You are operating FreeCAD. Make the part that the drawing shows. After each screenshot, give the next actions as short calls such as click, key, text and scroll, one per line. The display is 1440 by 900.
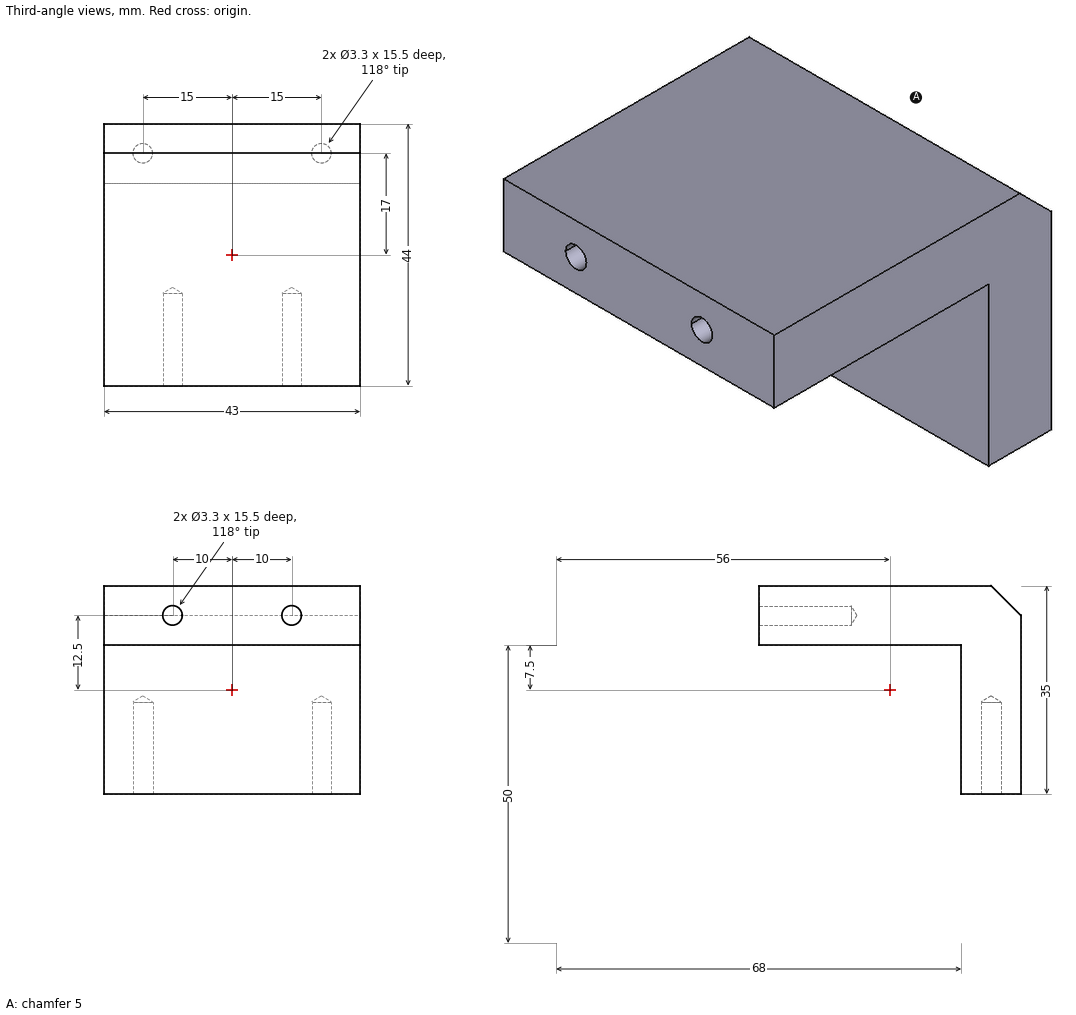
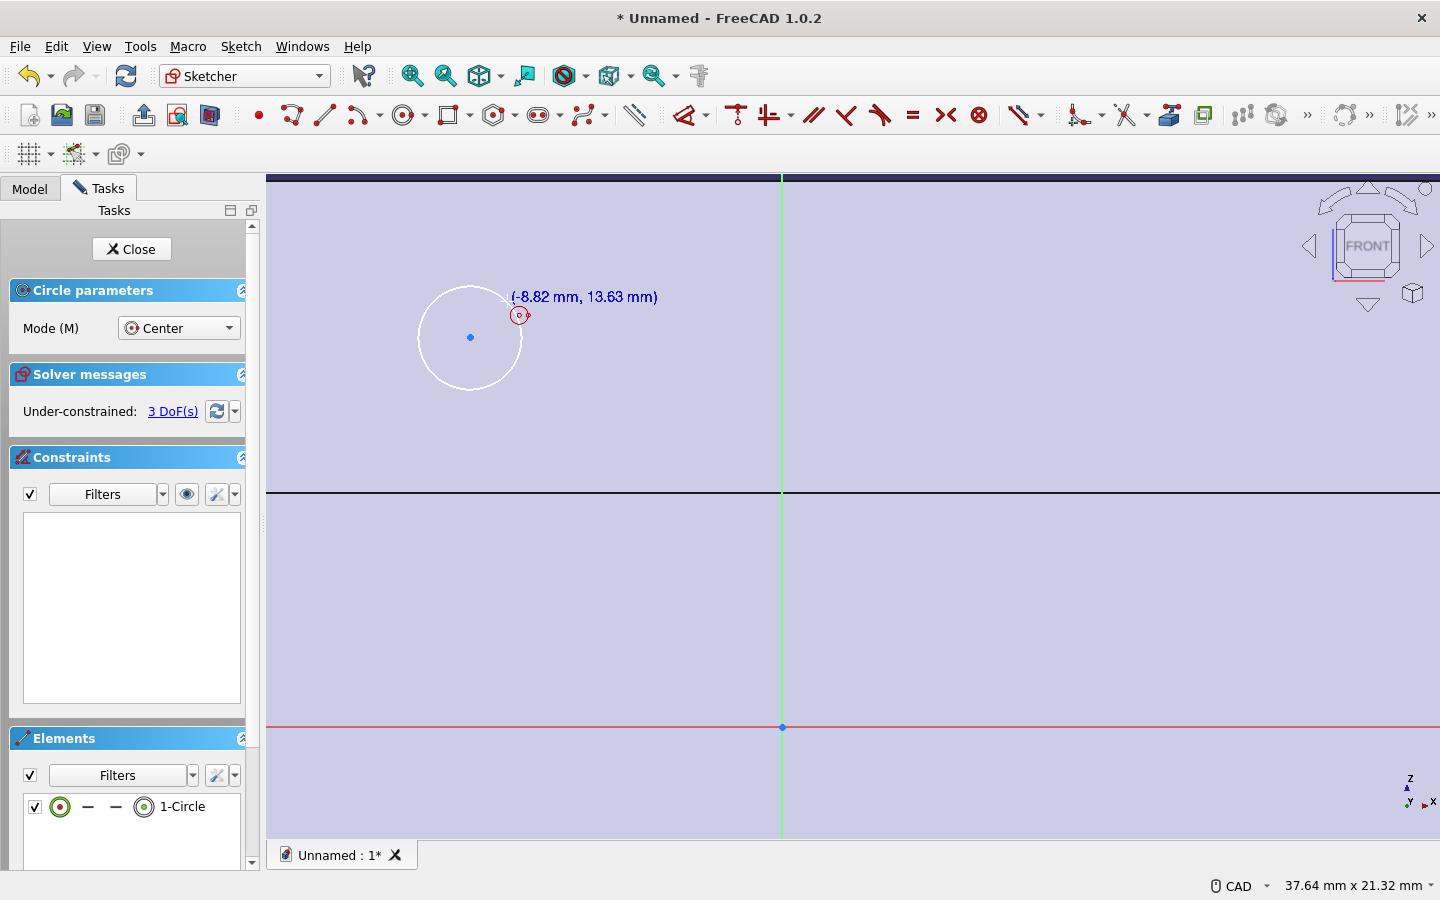
click(1094, 337)
click(1130, 301)
key(Escape)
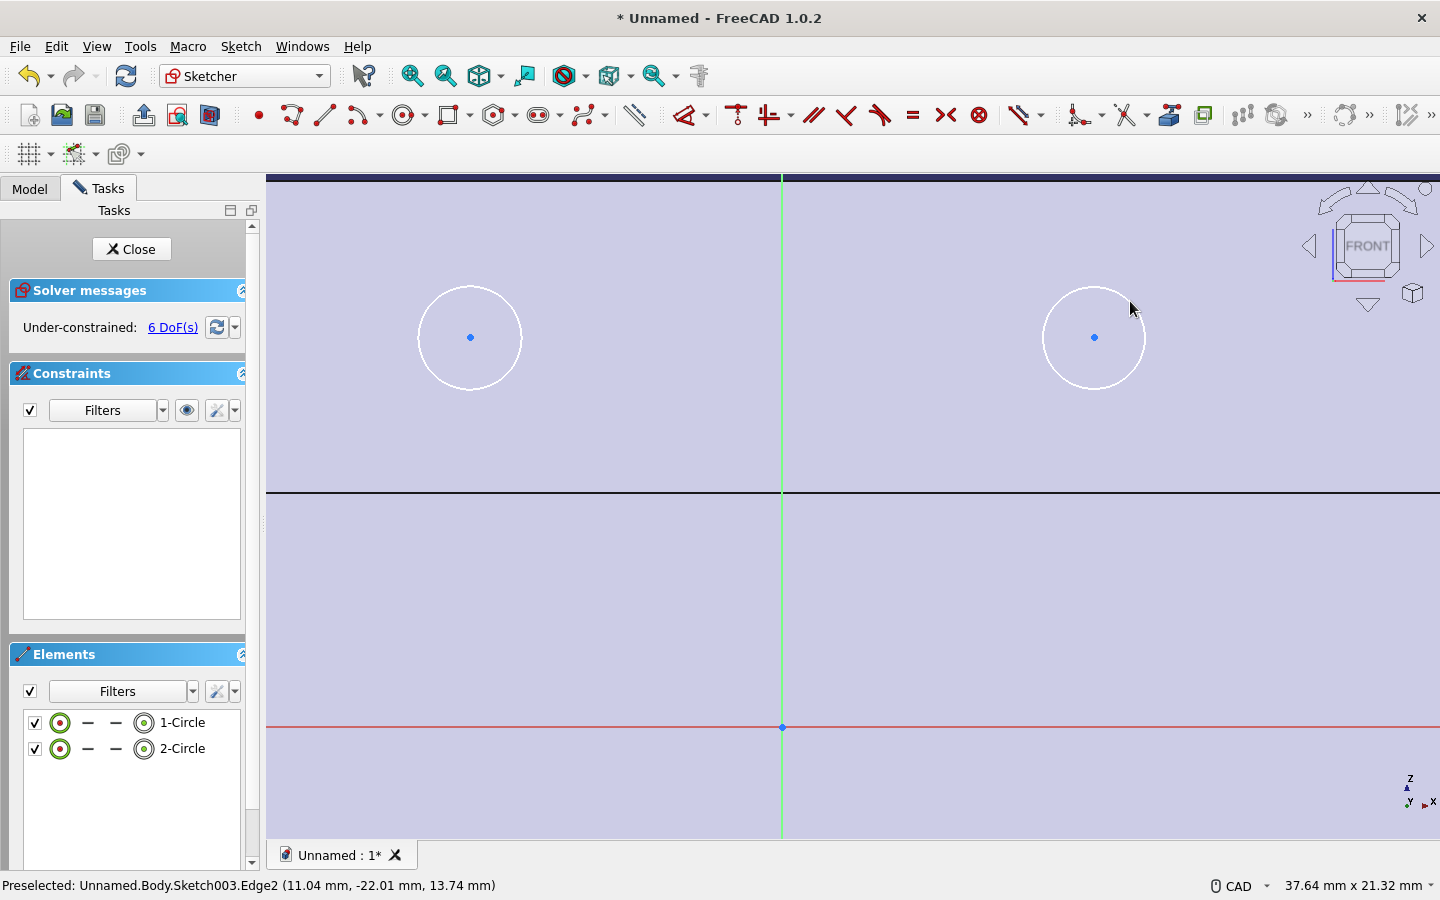
click(506, 301)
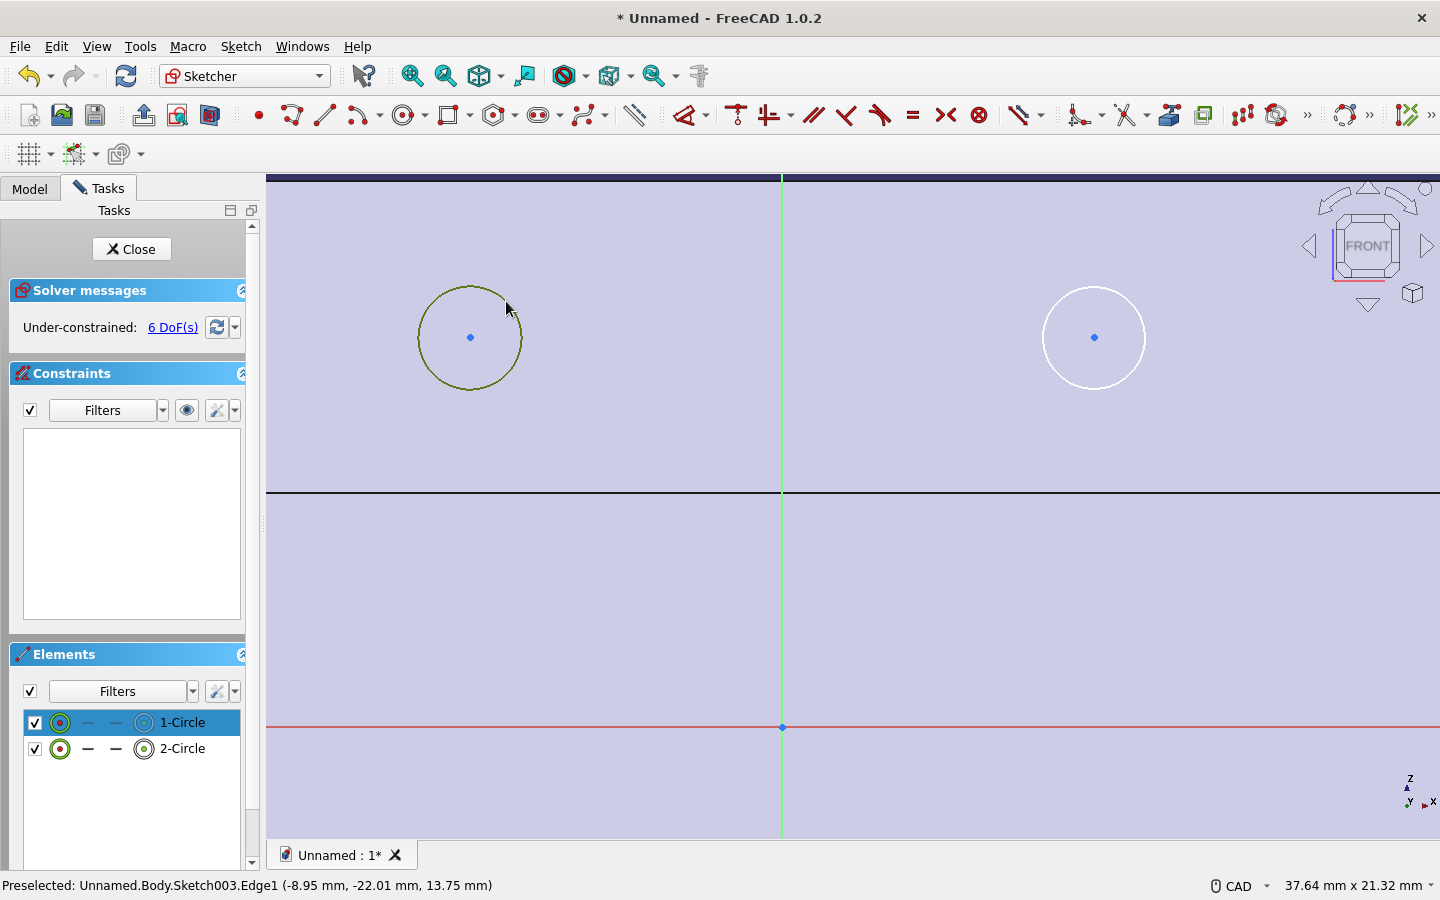
click(1130, 302)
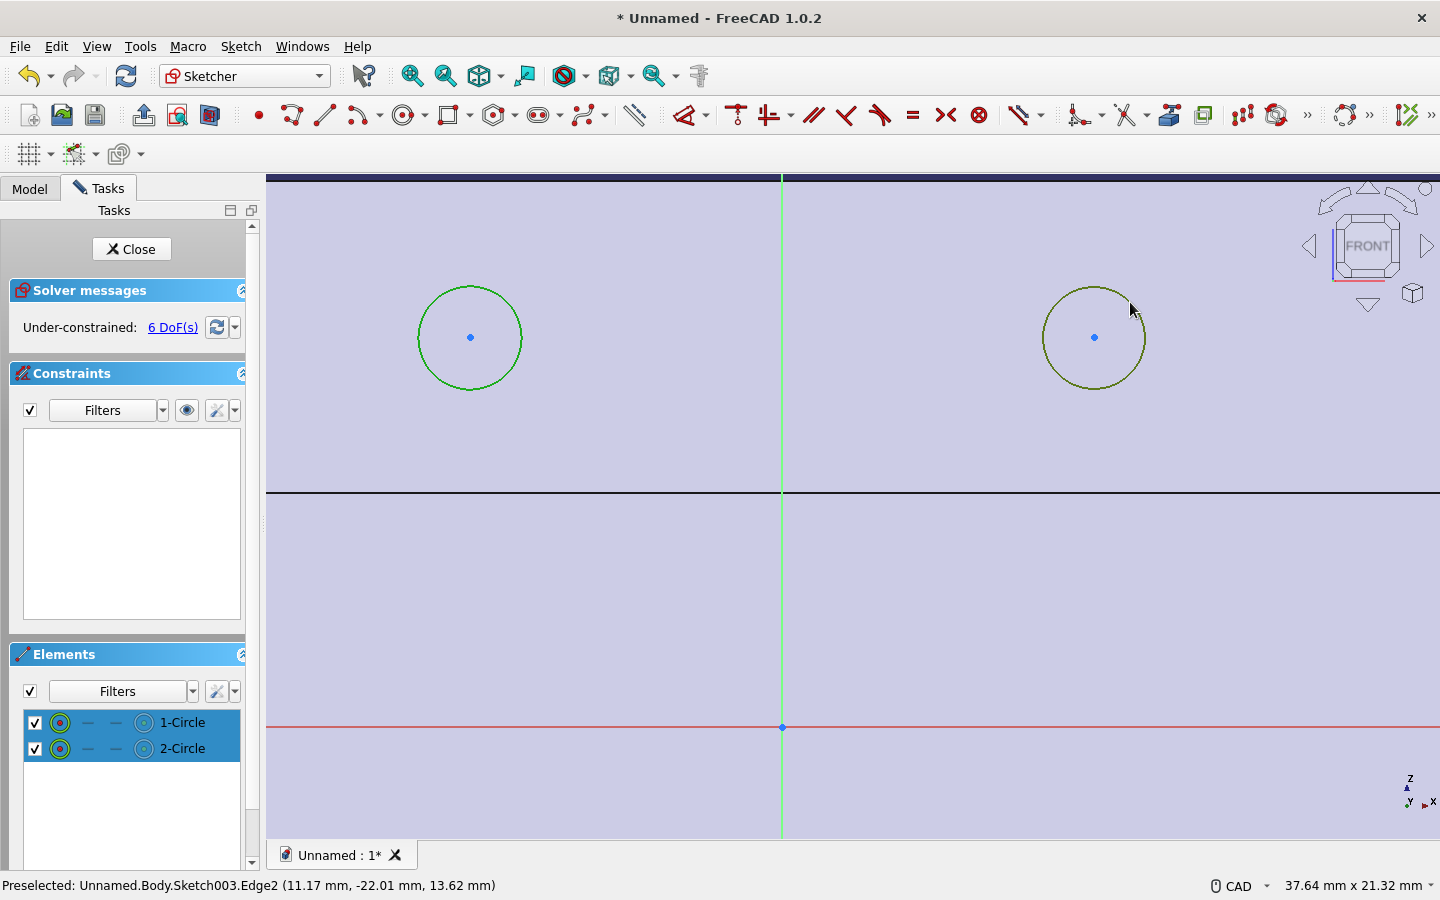
click(913, 116)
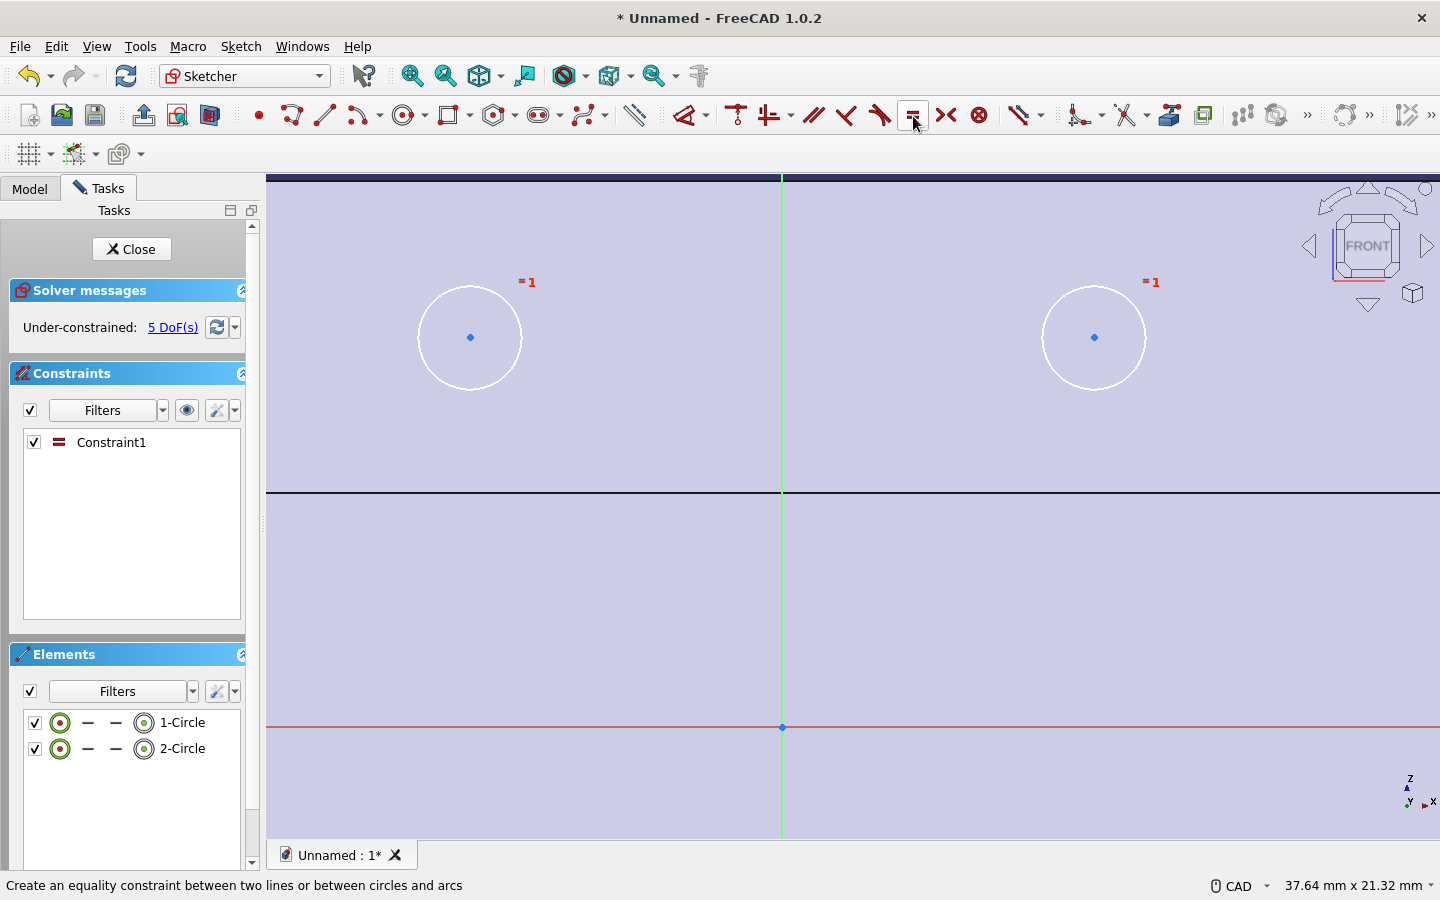
click(684, 116)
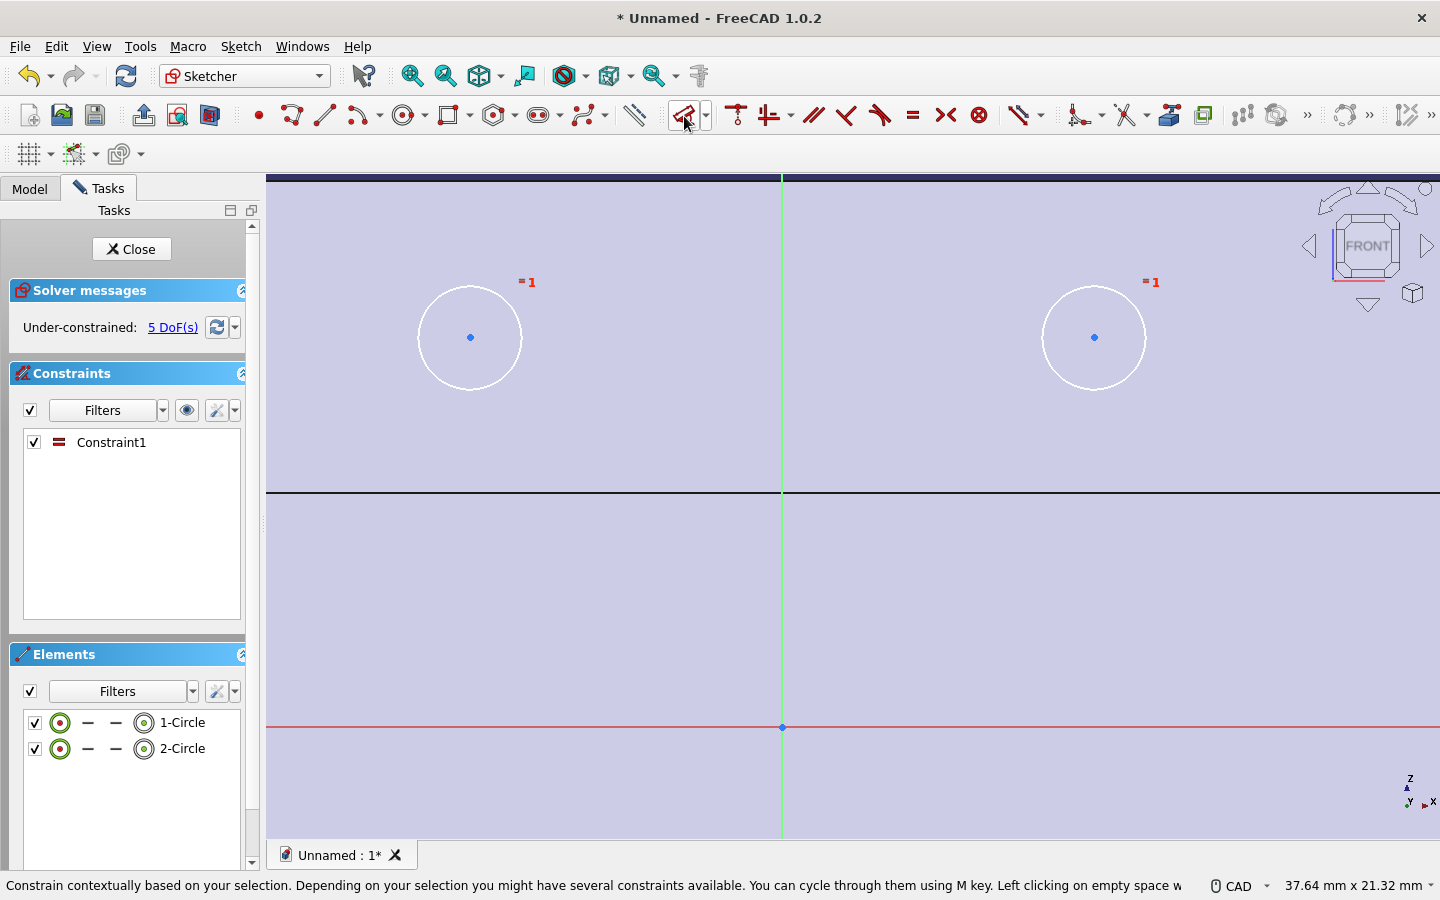
click(506, 301)
click(528, 278)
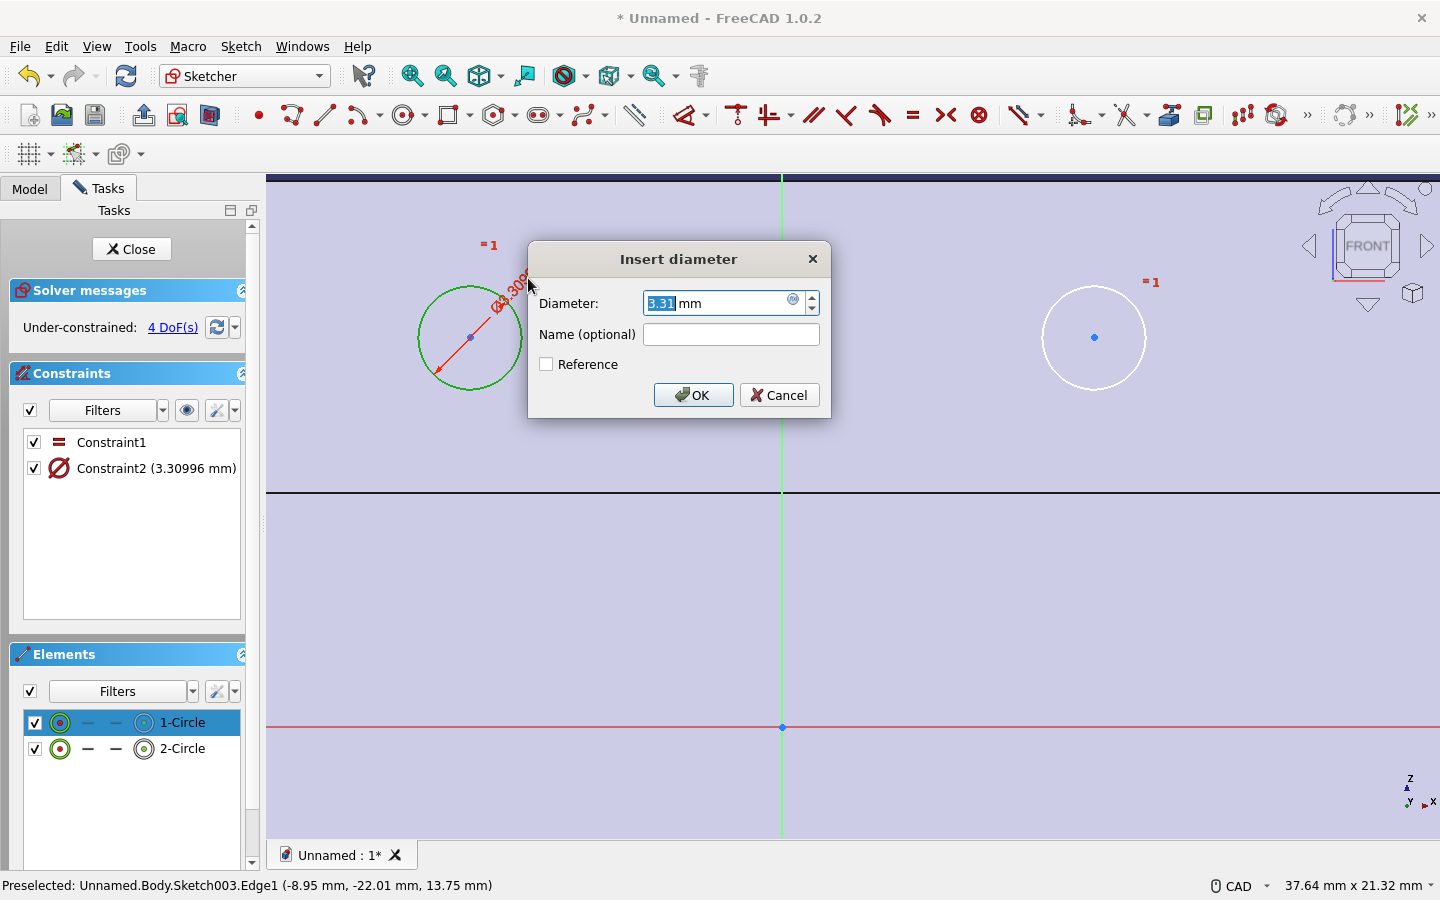
text(3.3)
key(Return)